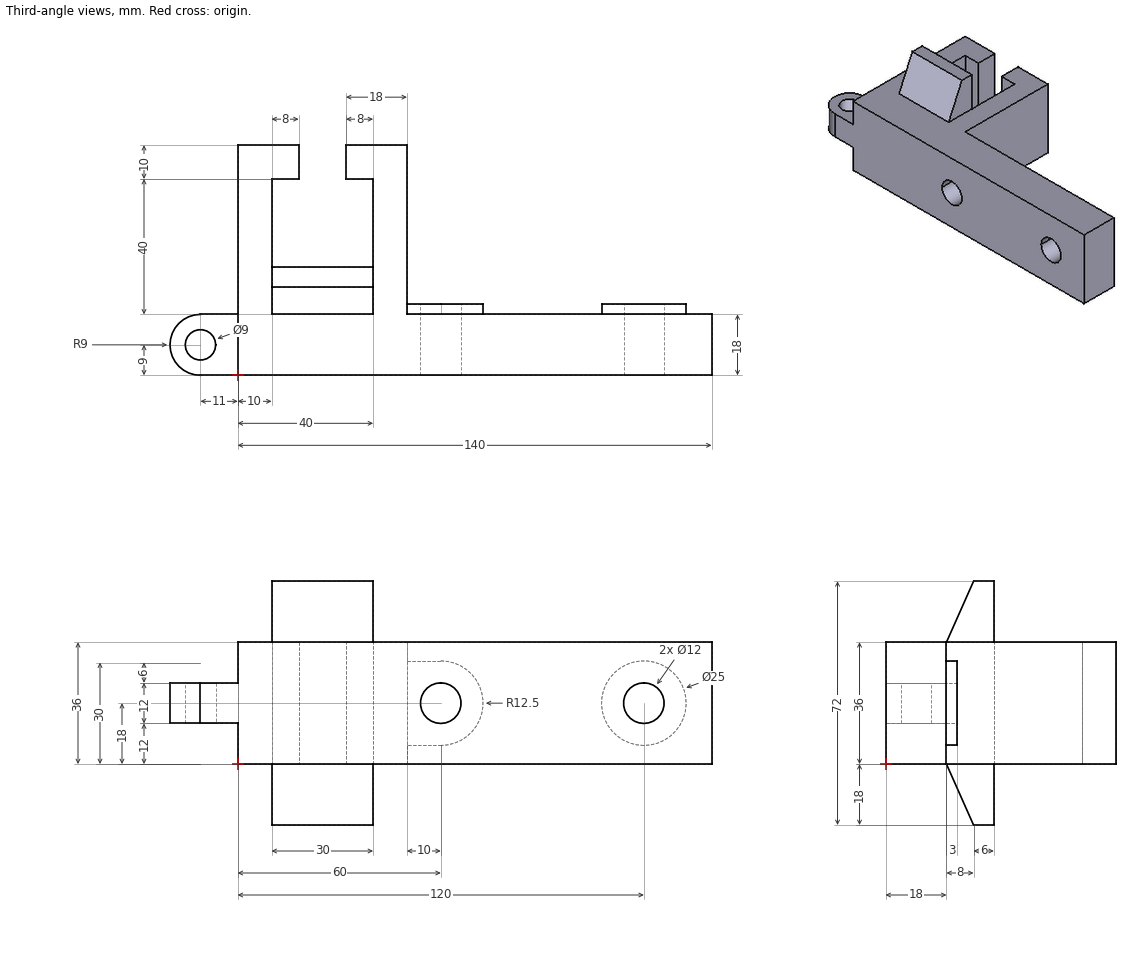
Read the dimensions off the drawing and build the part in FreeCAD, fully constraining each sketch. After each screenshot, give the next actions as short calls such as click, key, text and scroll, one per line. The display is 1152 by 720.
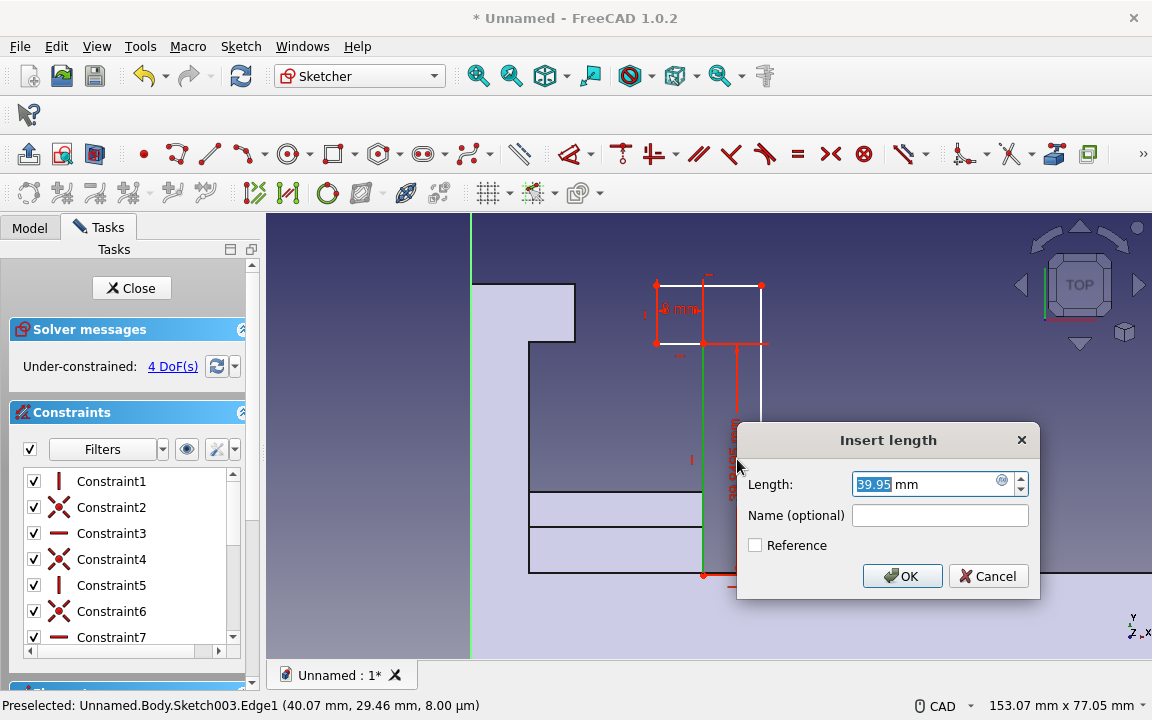
text(40)
key(Return)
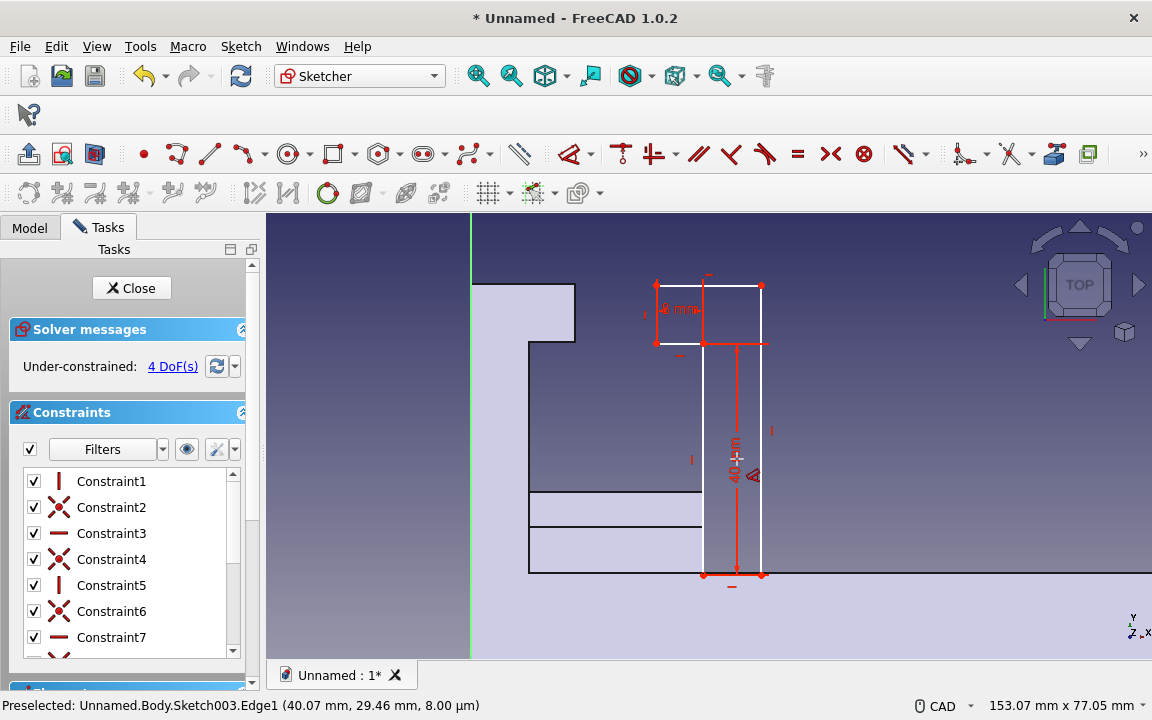
click(657, 326)
click(623, 335)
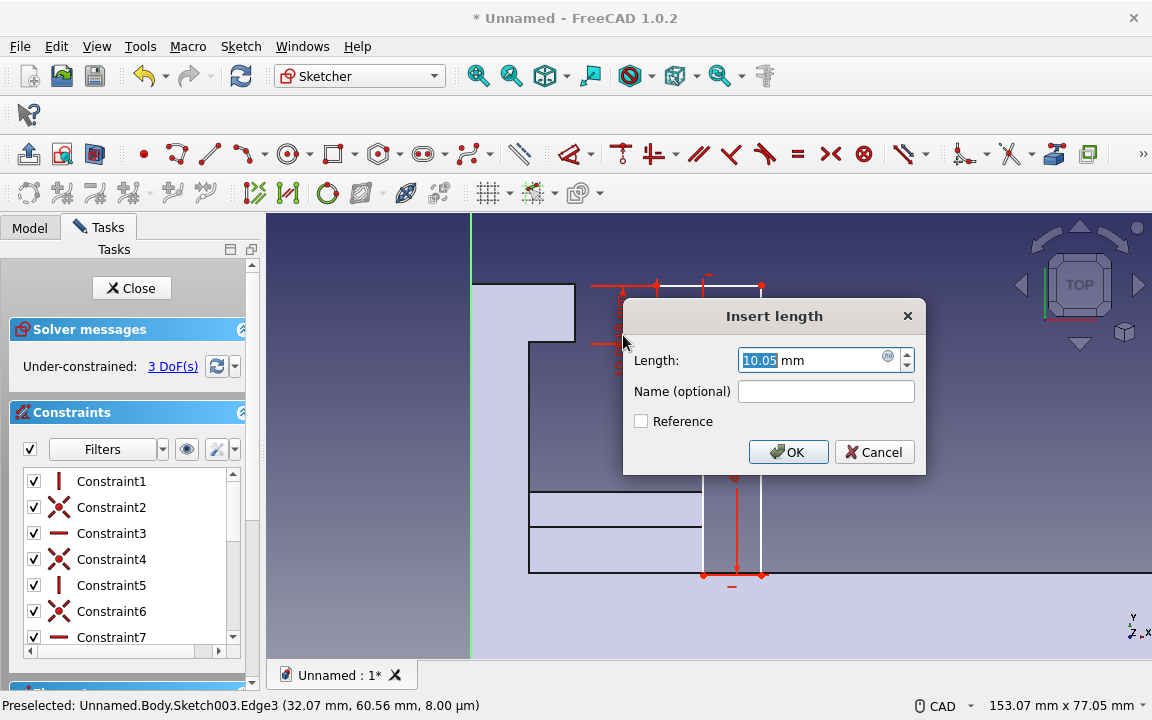
text(10)
key(Return)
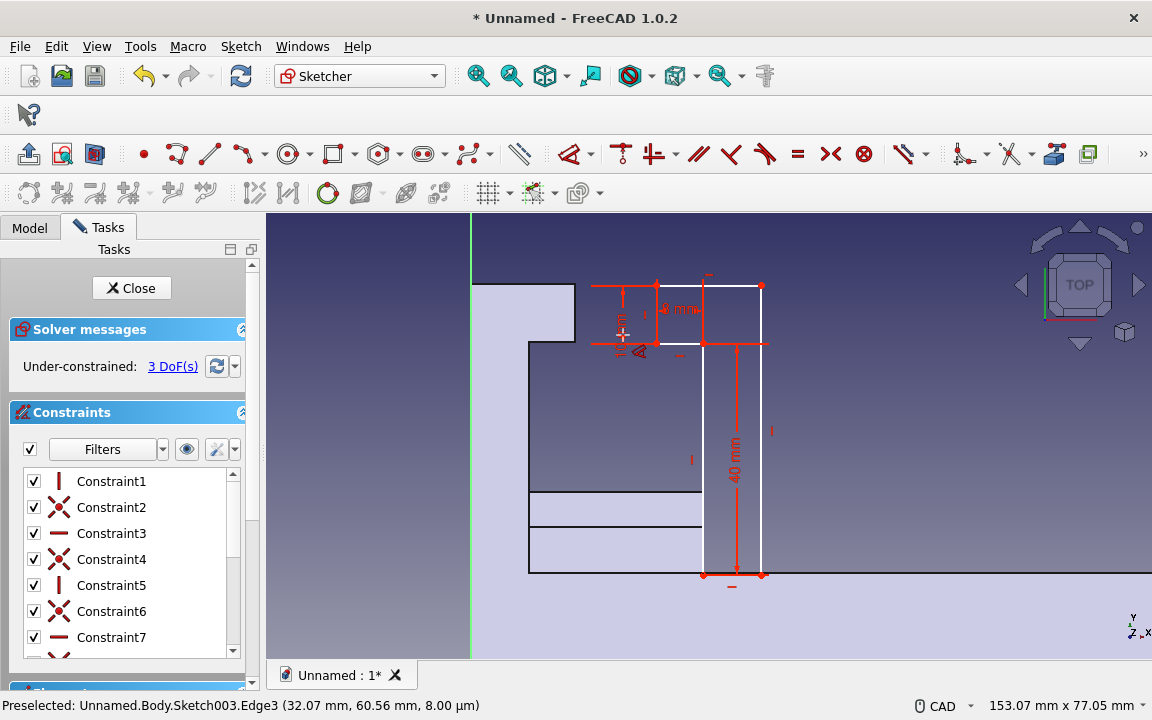
click(688, 286)
click(709, 252)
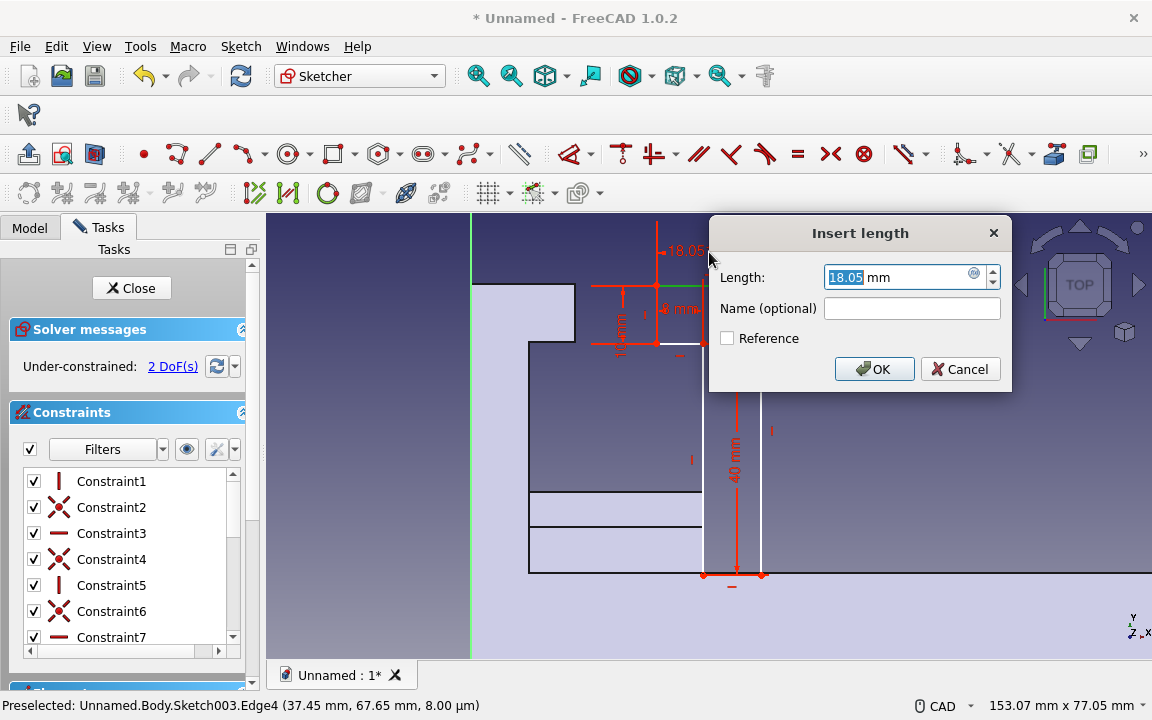
text(18)
key(Return)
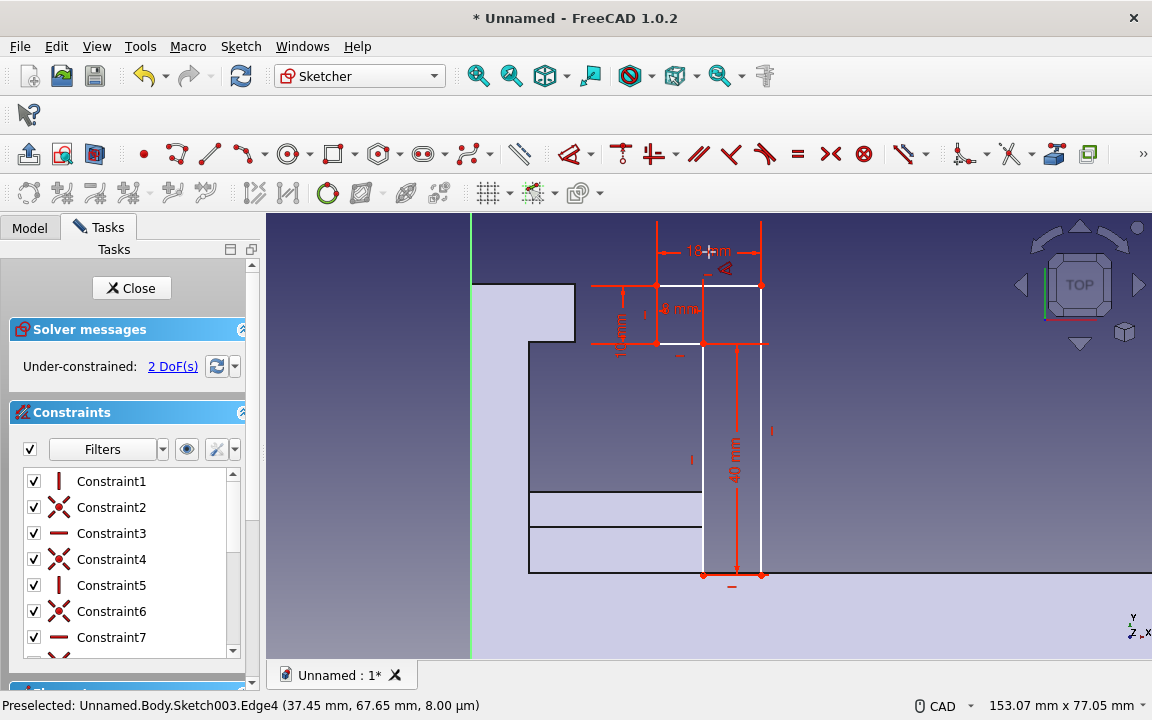
click(703, 575)
click(587, 541)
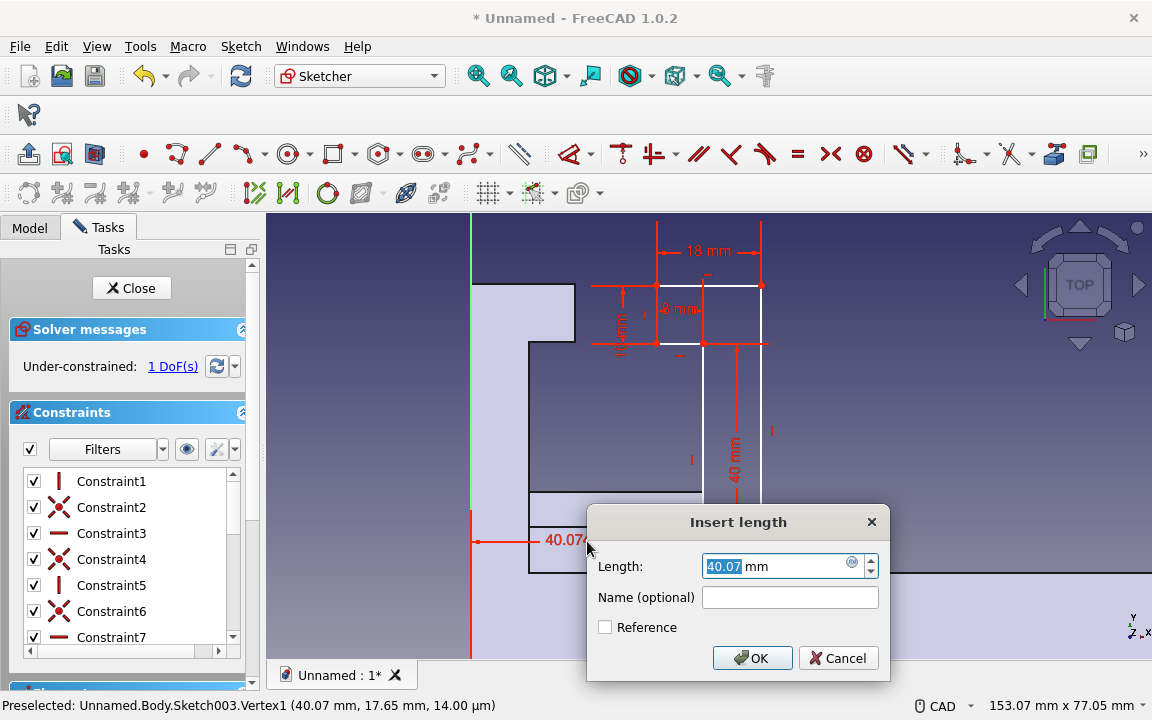
text(40)
key(Return)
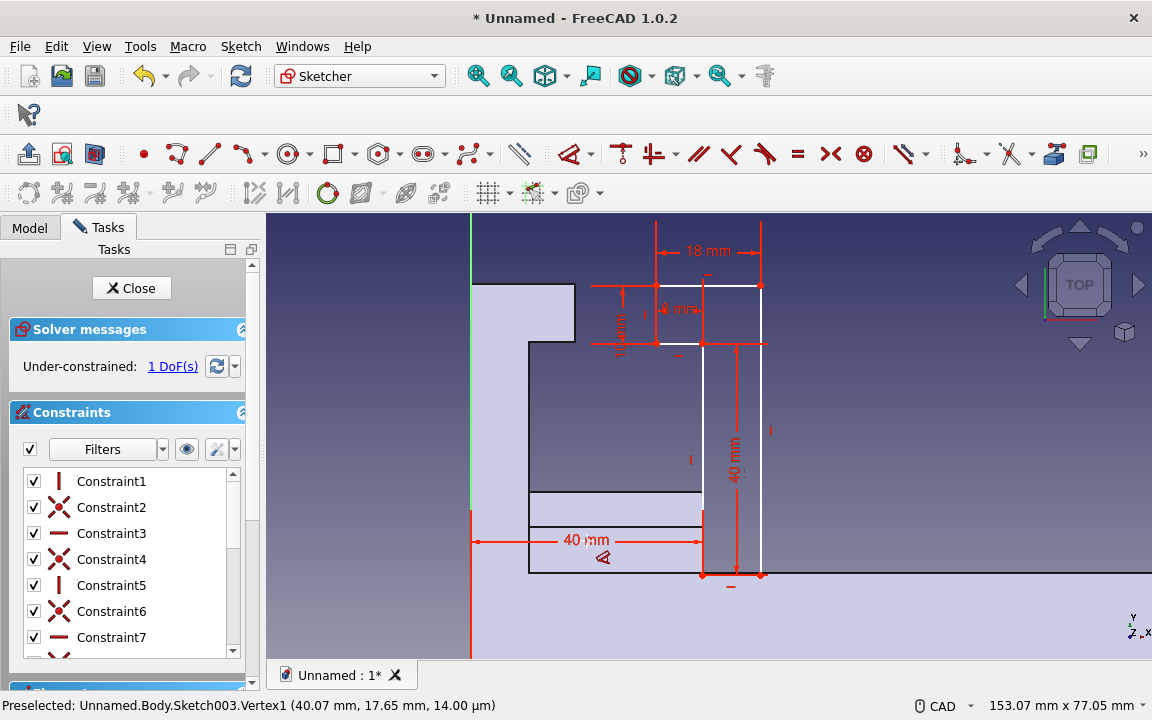
click(703, 575)
click(437, 603)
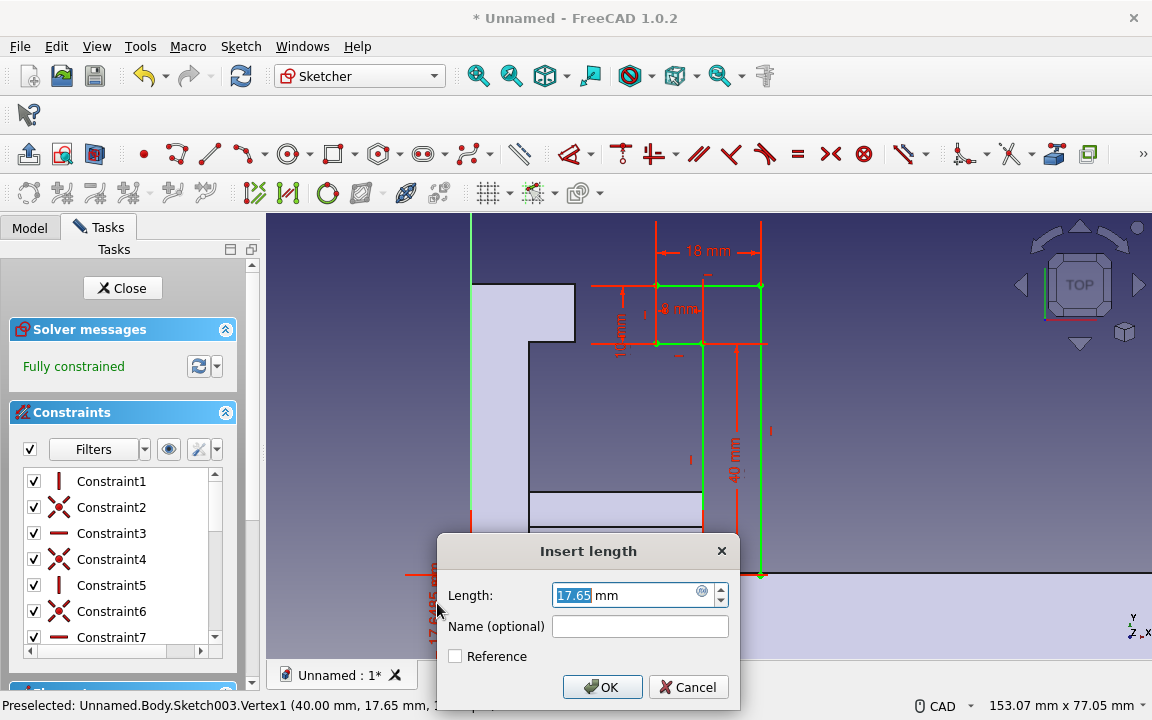
text(18)
key(Return)
key(Escape)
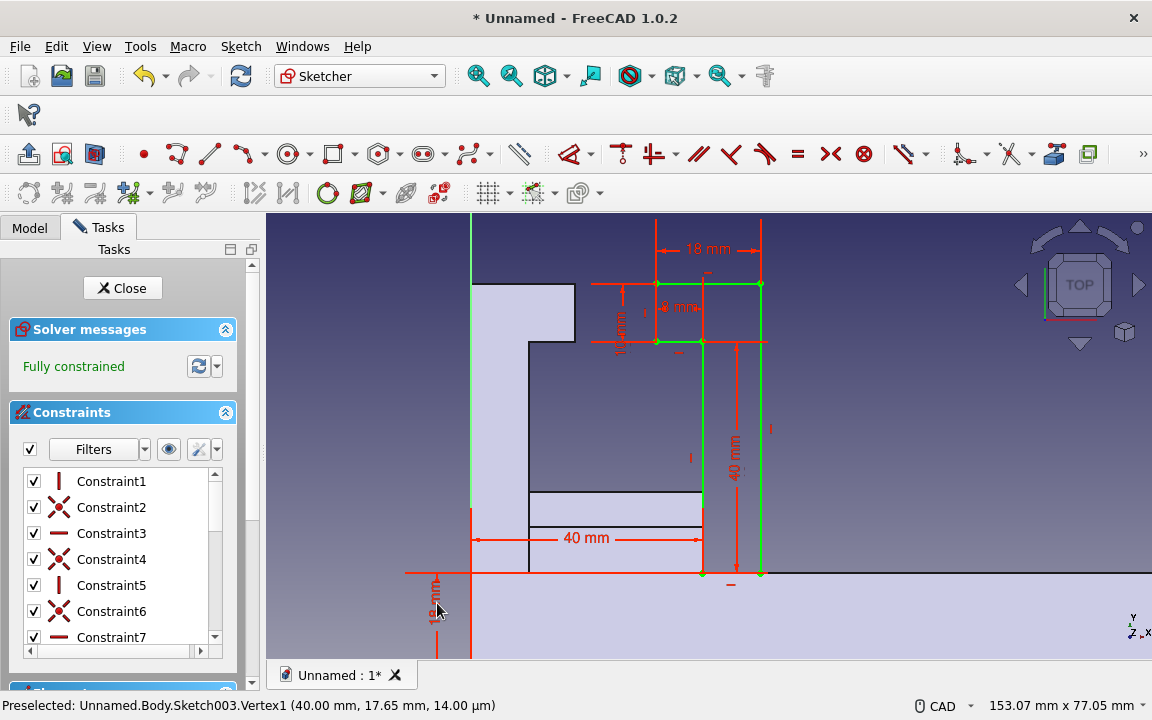
click(123, 288)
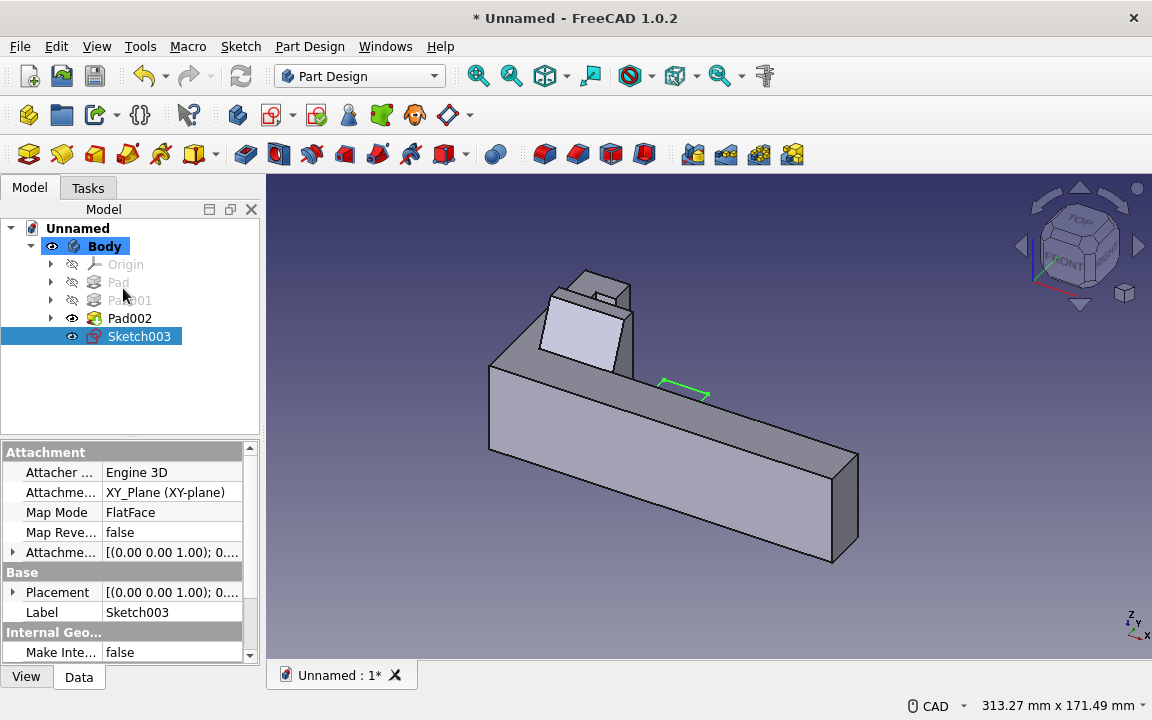
click(29, 154)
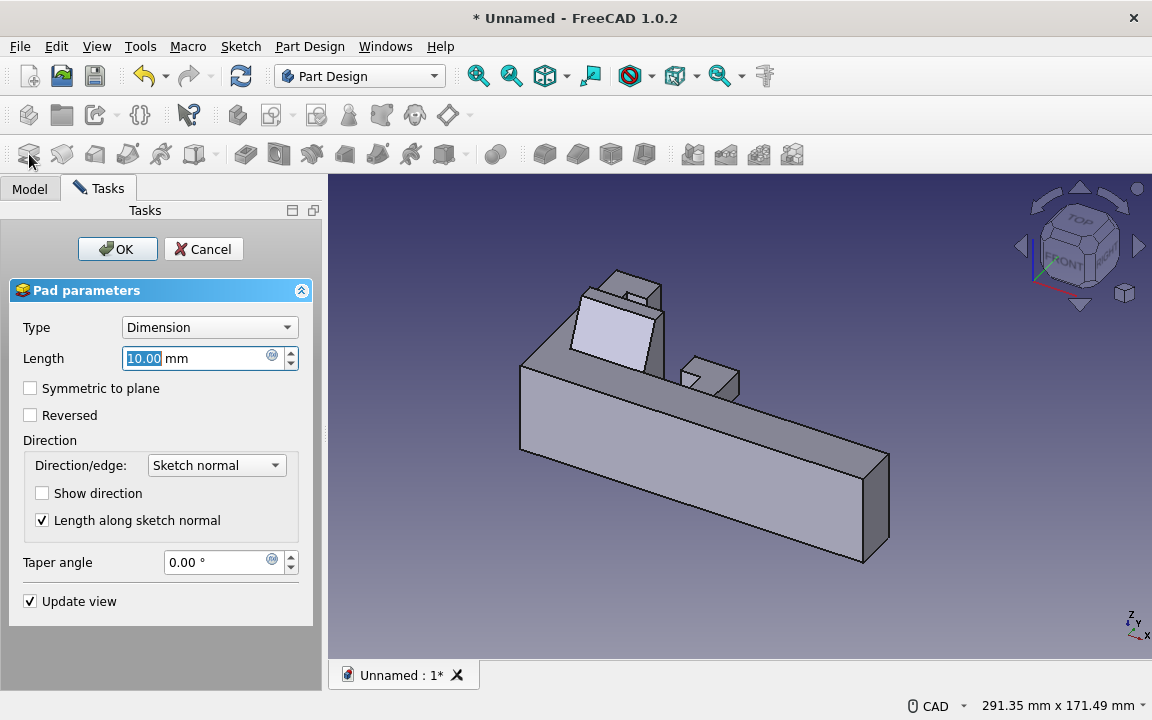
text(36)
key(Tab)